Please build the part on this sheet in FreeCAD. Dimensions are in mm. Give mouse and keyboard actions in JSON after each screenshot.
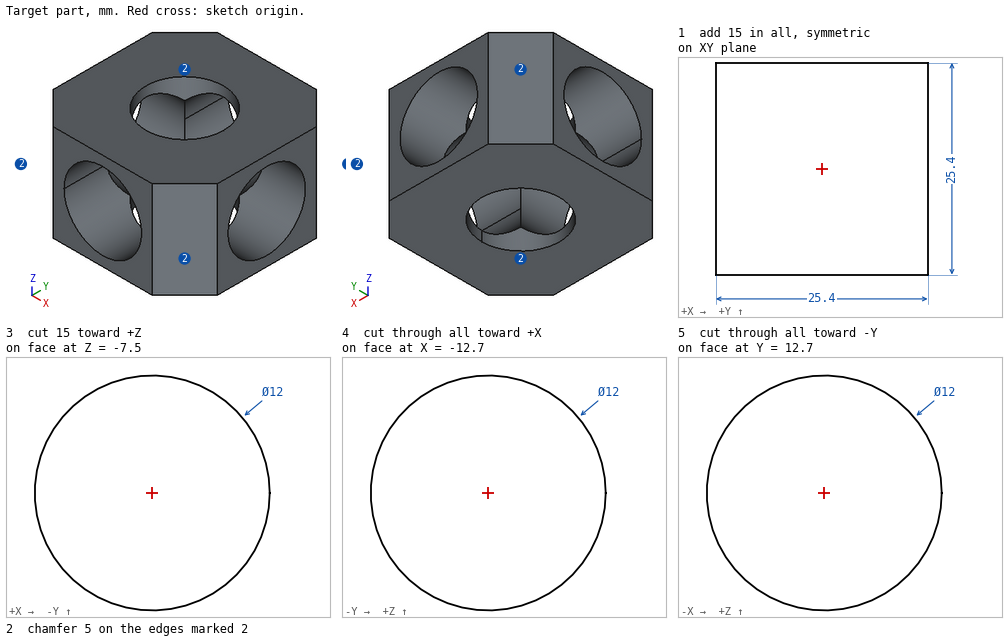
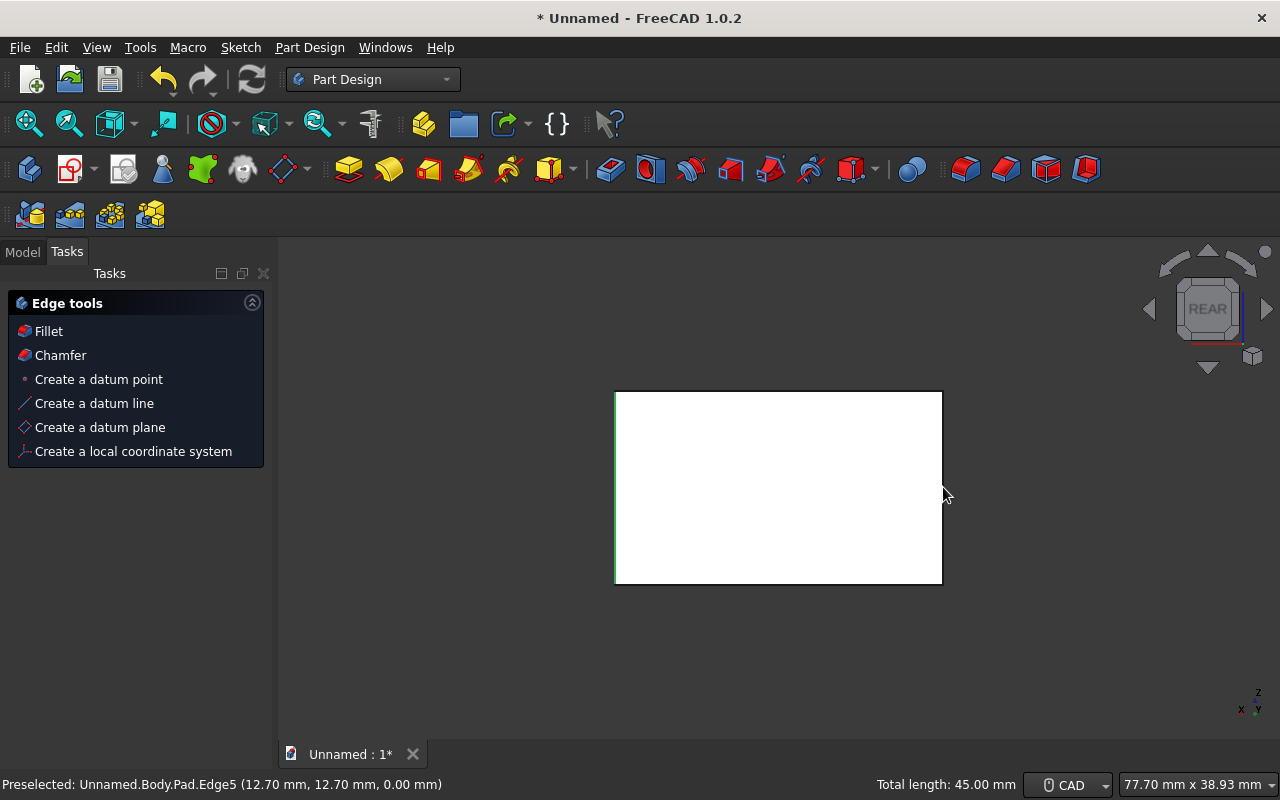
{"action": "left_click", "coordinate": [943, 487], "text": "ctrl"}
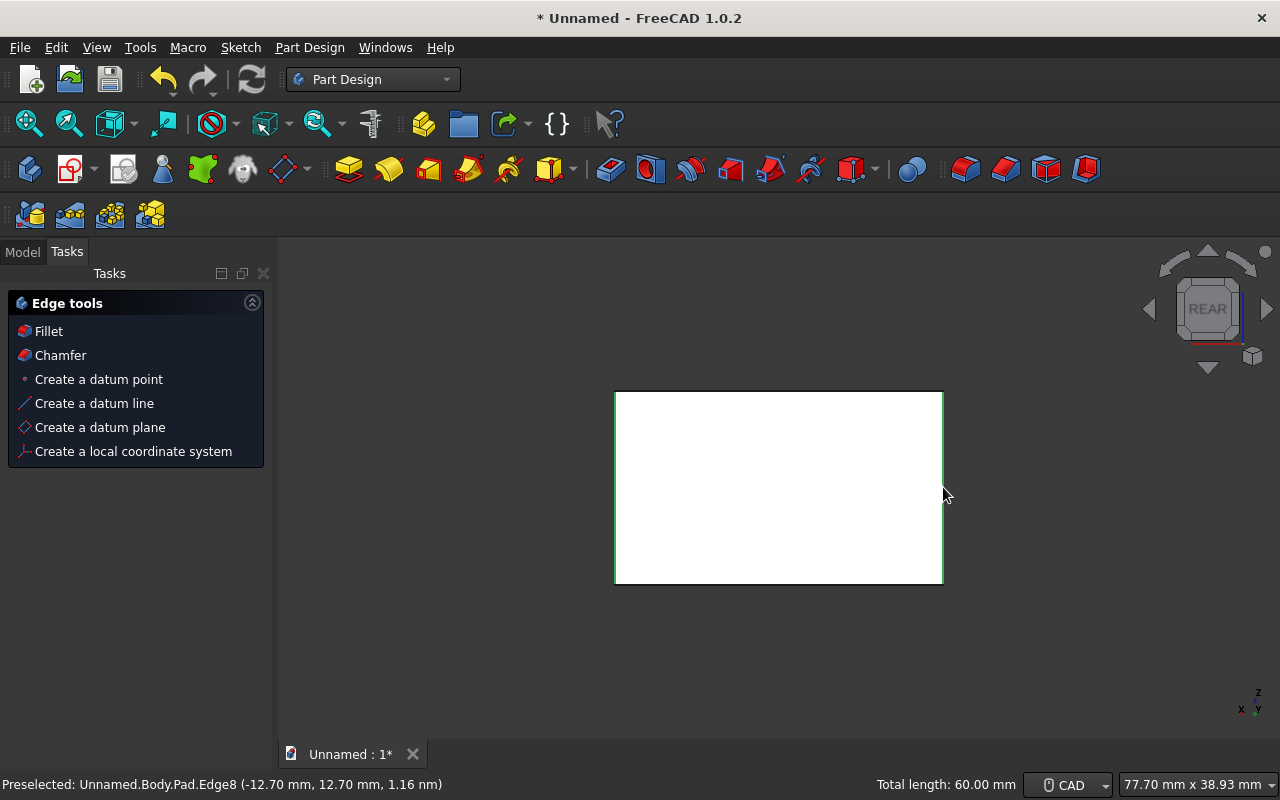
{"action": "left_click", "coordinate": [1006, 170]}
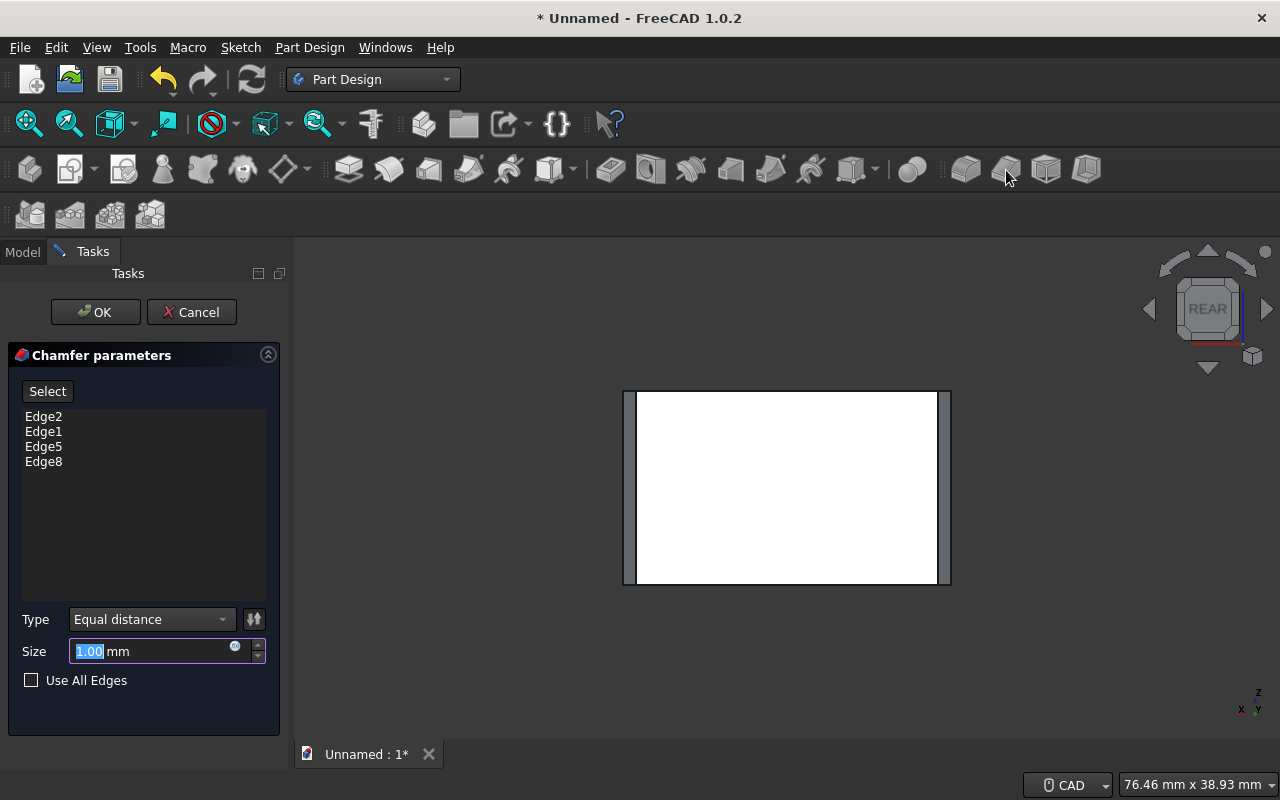
{"action": "type", "text": "5"}
{"action": "key", "text": "Tab"}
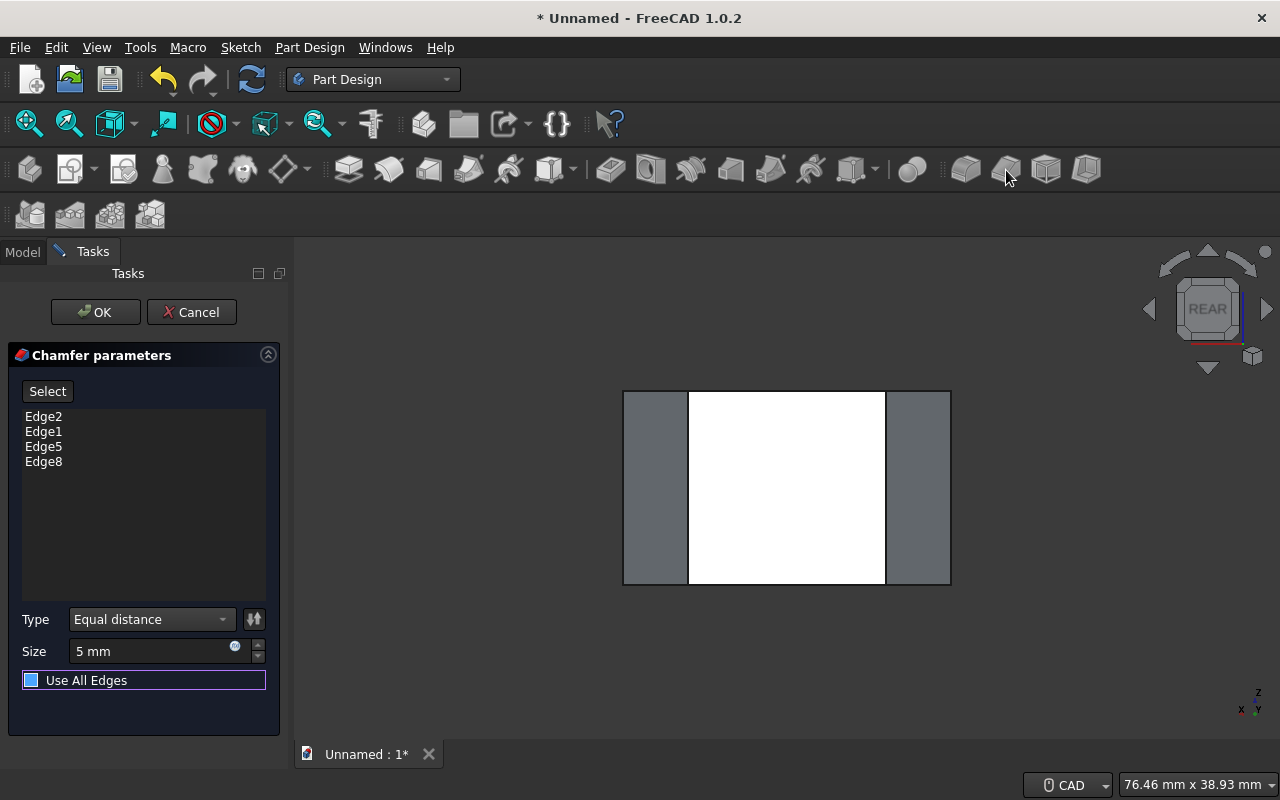
{"action": "left_click", "coordinate": [96, 312]}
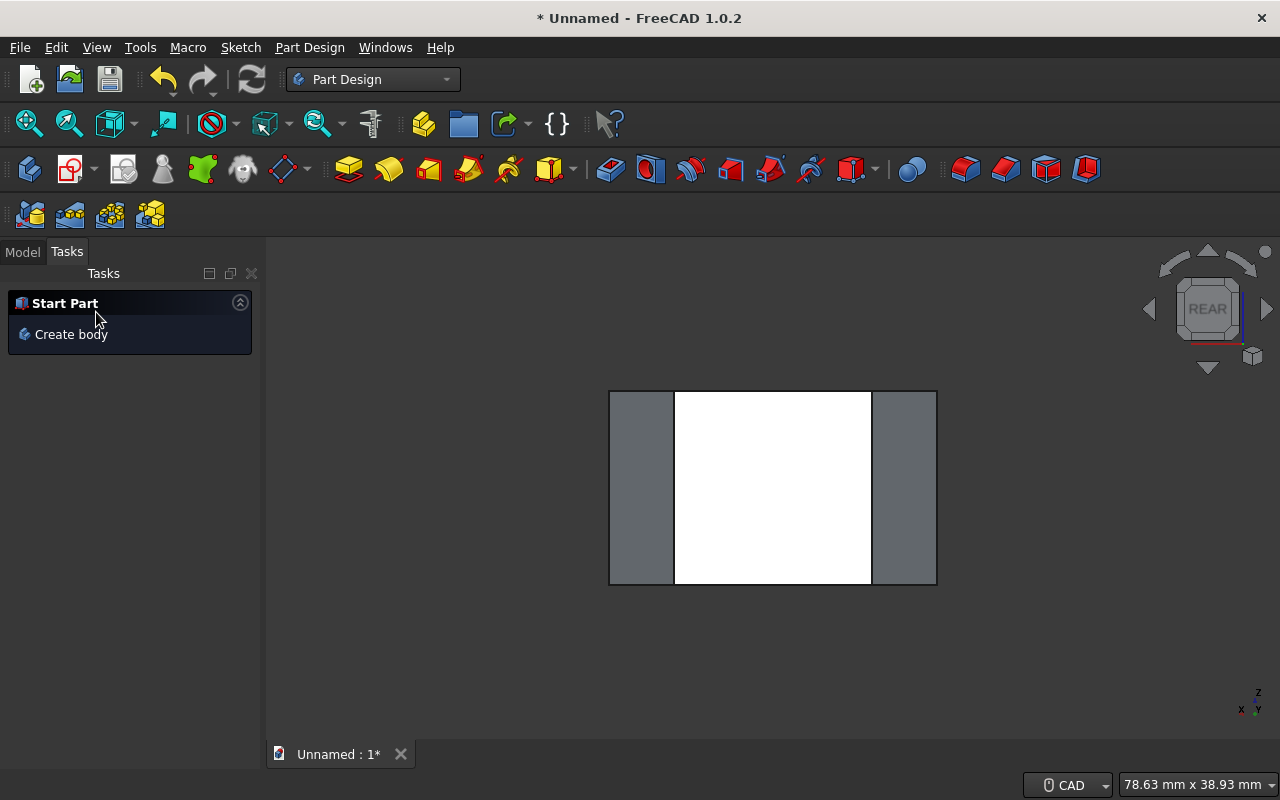
{"action": "key", "text": "v f"}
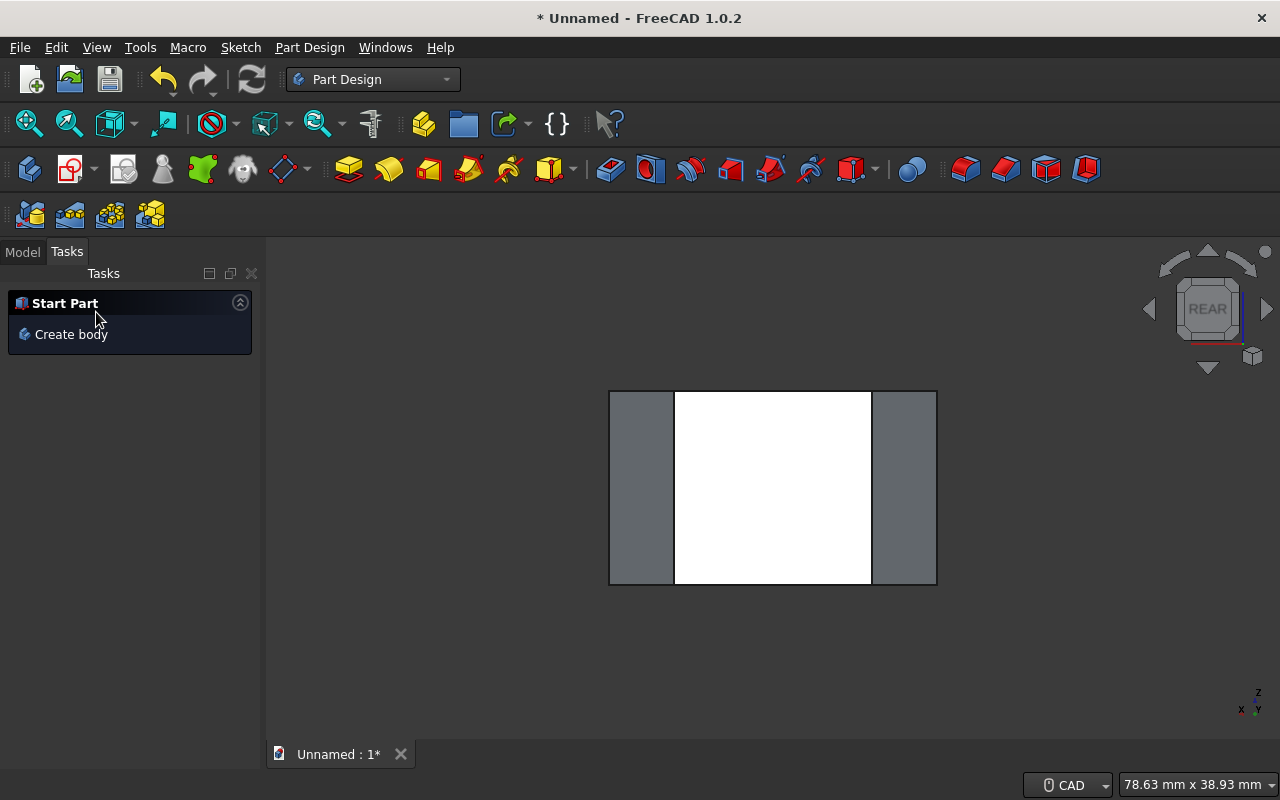
{"action": "key", "text": "5"}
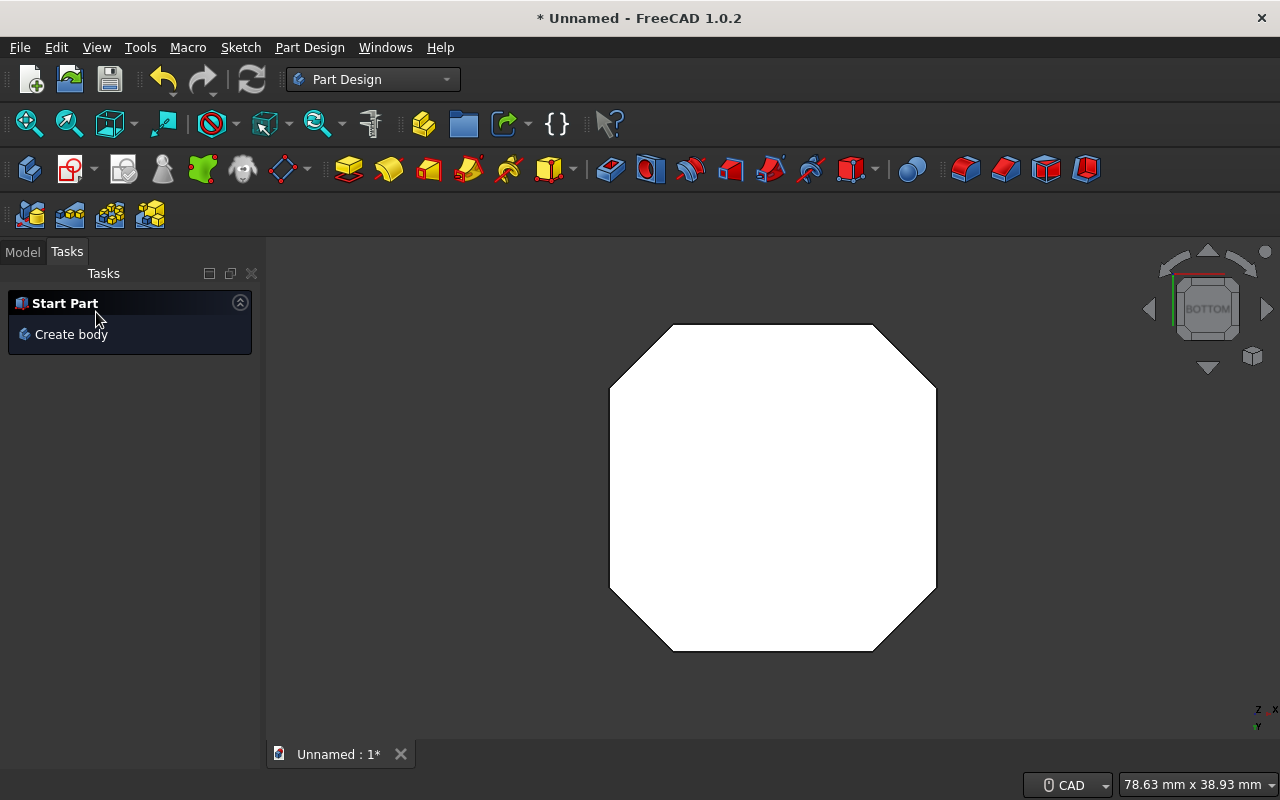
{"action": "left_click", "coordinate": [773, 487]}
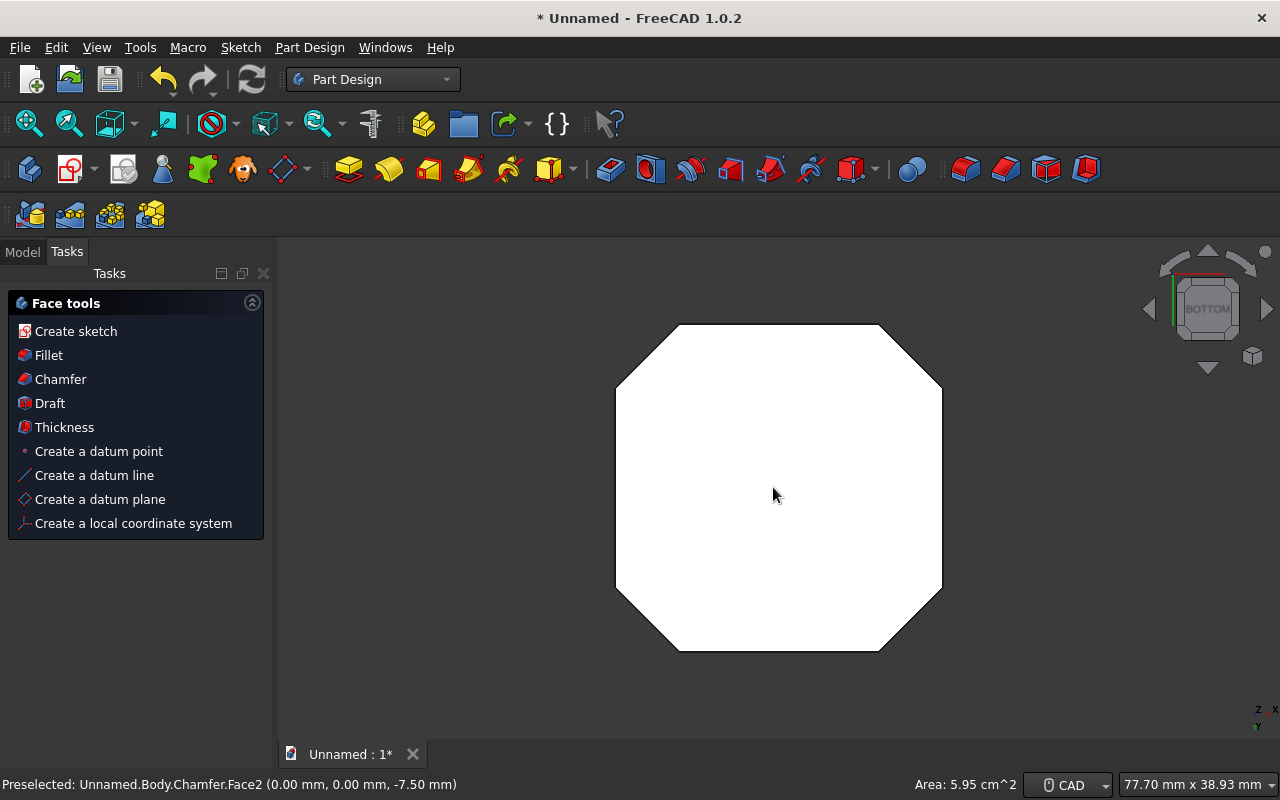
{"action": "left_click", "coordinate": [70, 170]}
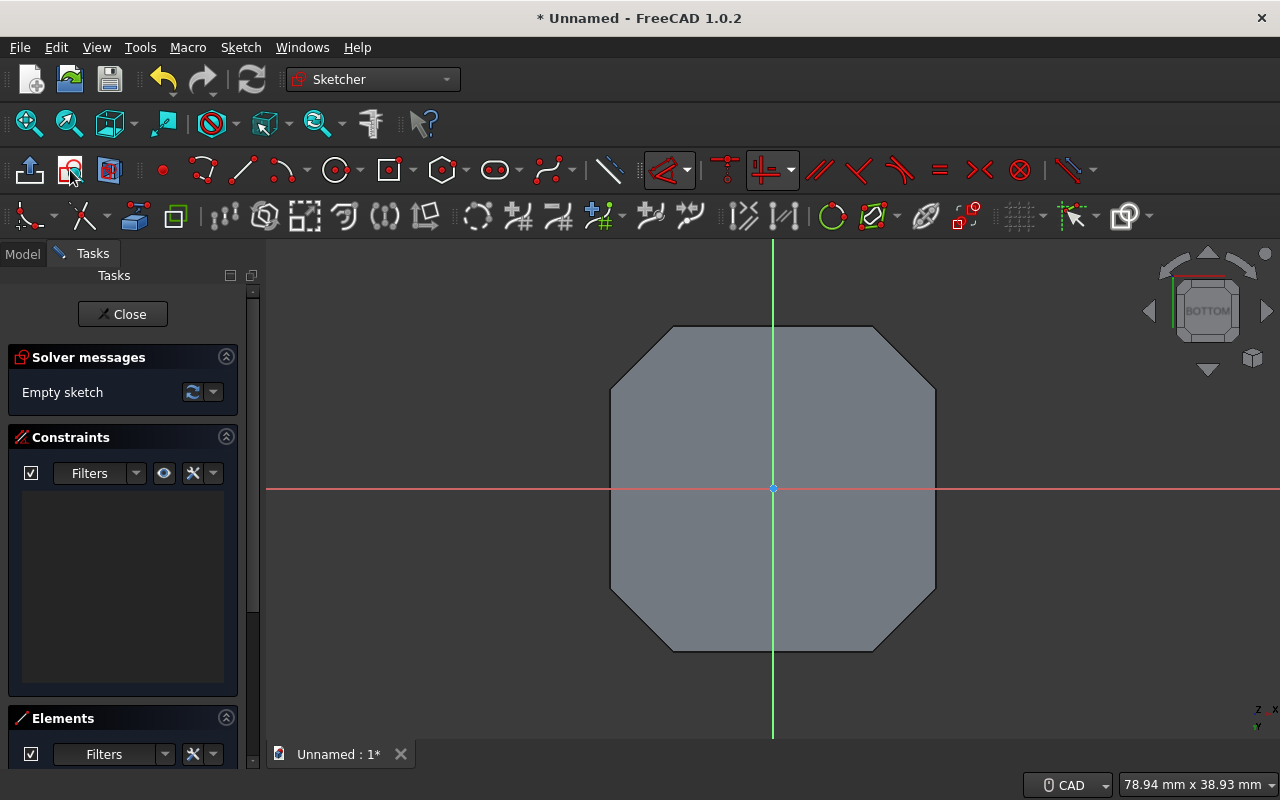
{"action": "scroll", "coordinate": [829, 489], "scroll_direction": "up", "scroll_amount": 4}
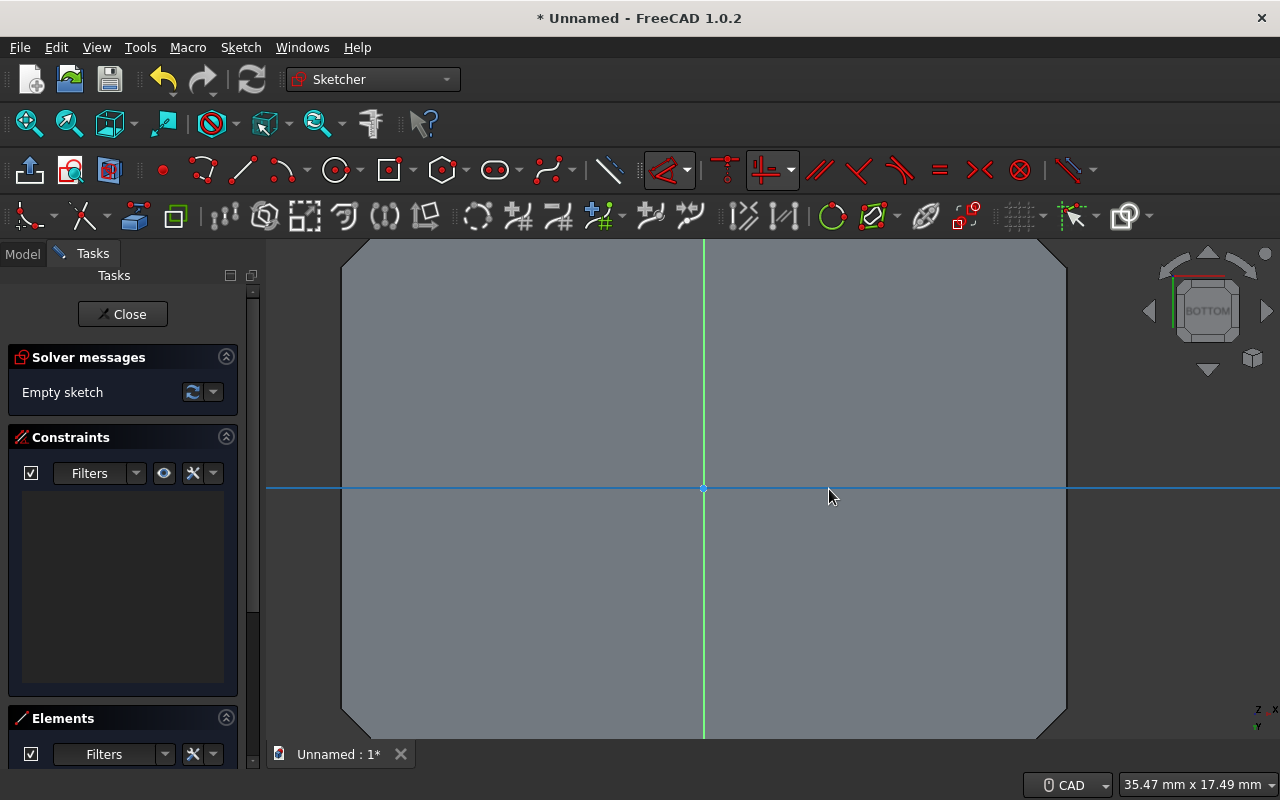
{"action": "left_click", "coordinate": [336, 170]}